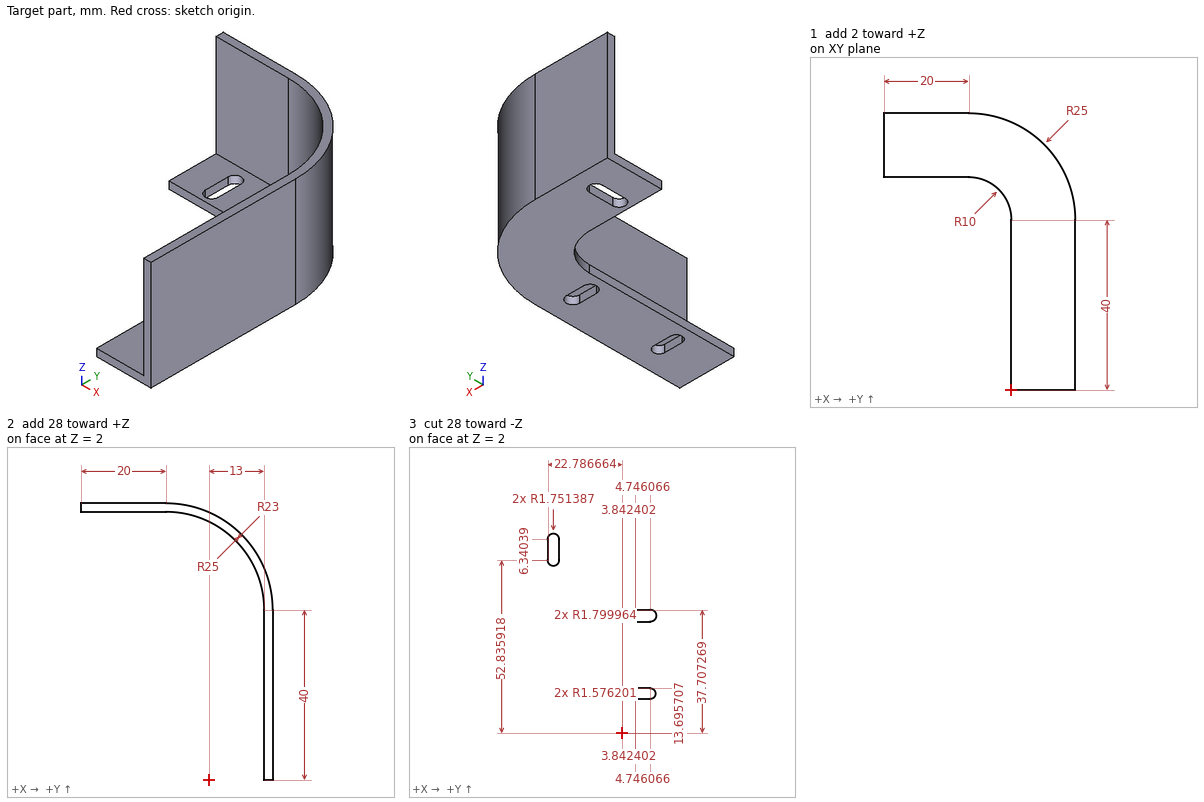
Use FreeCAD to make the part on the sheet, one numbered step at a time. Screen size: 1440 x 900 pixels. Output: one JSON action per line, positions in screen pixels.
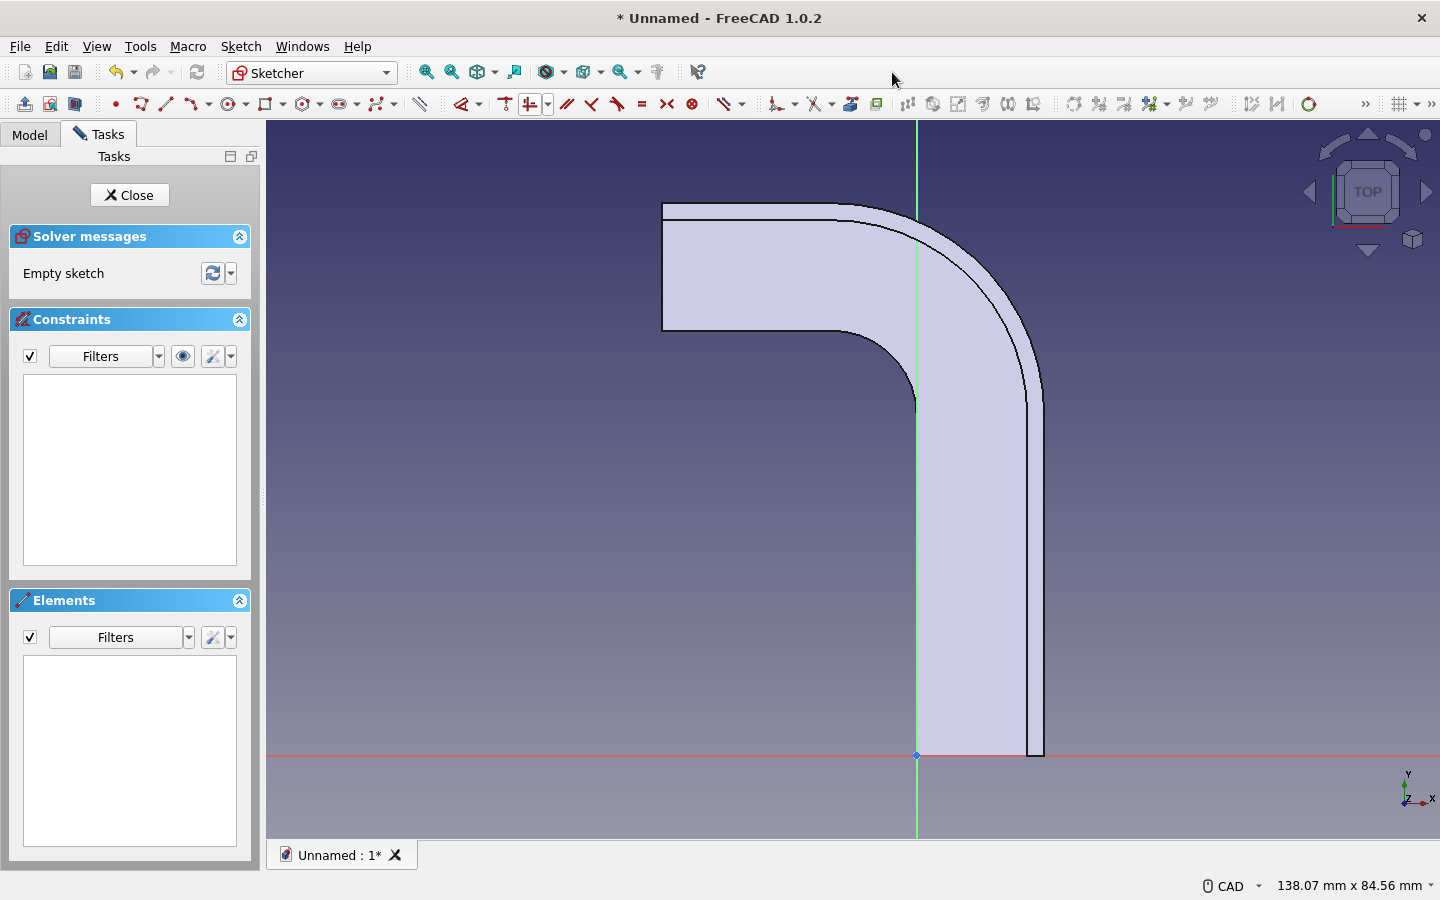
{"action": "left_click", "coordinate": [75, 104]}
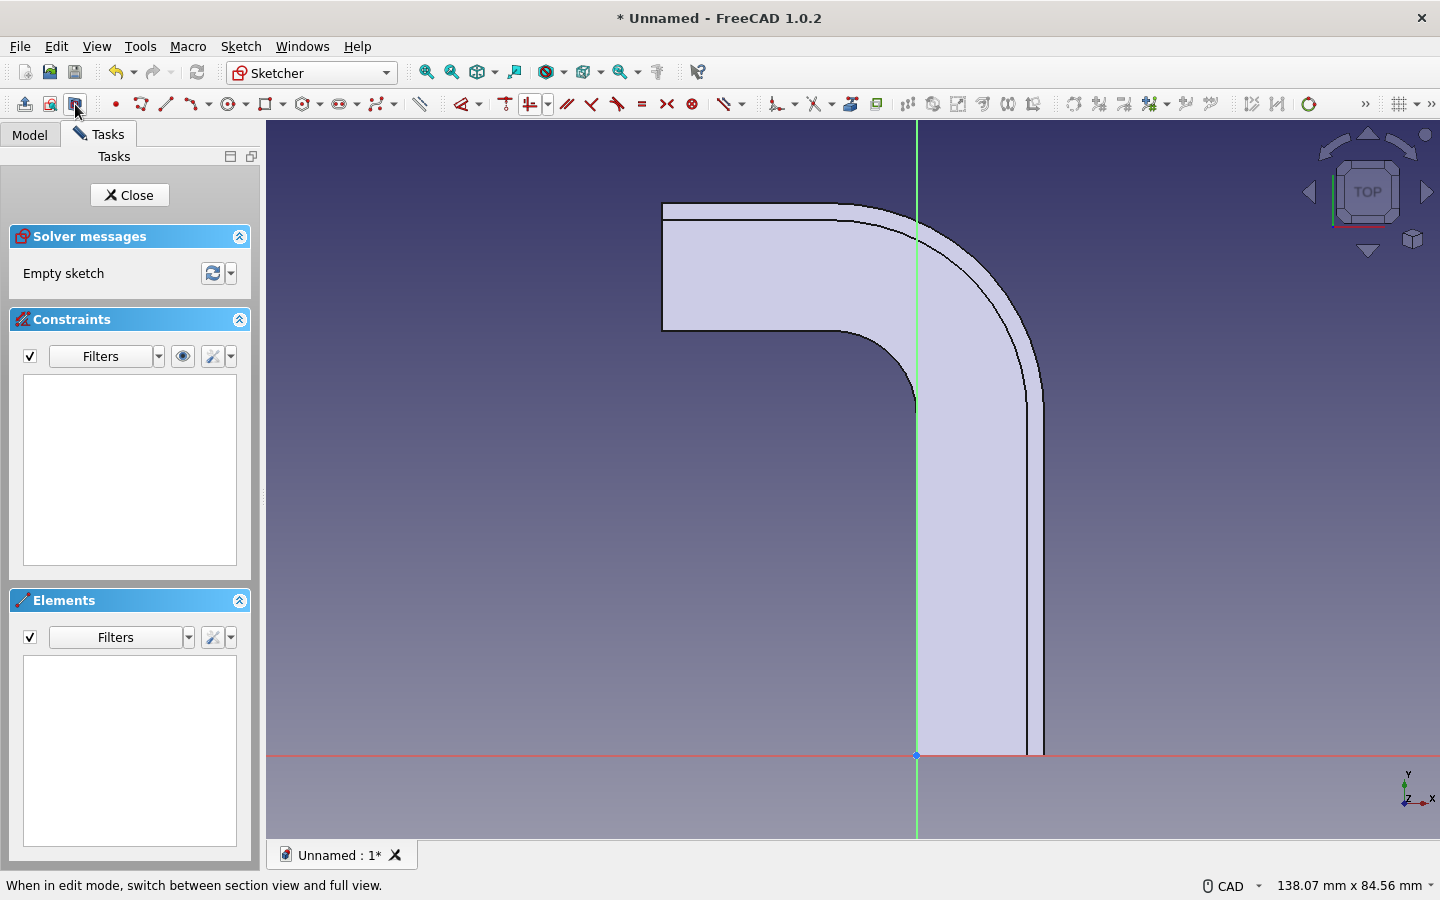
{"action": "left_click", "coordinate": [338, 104]}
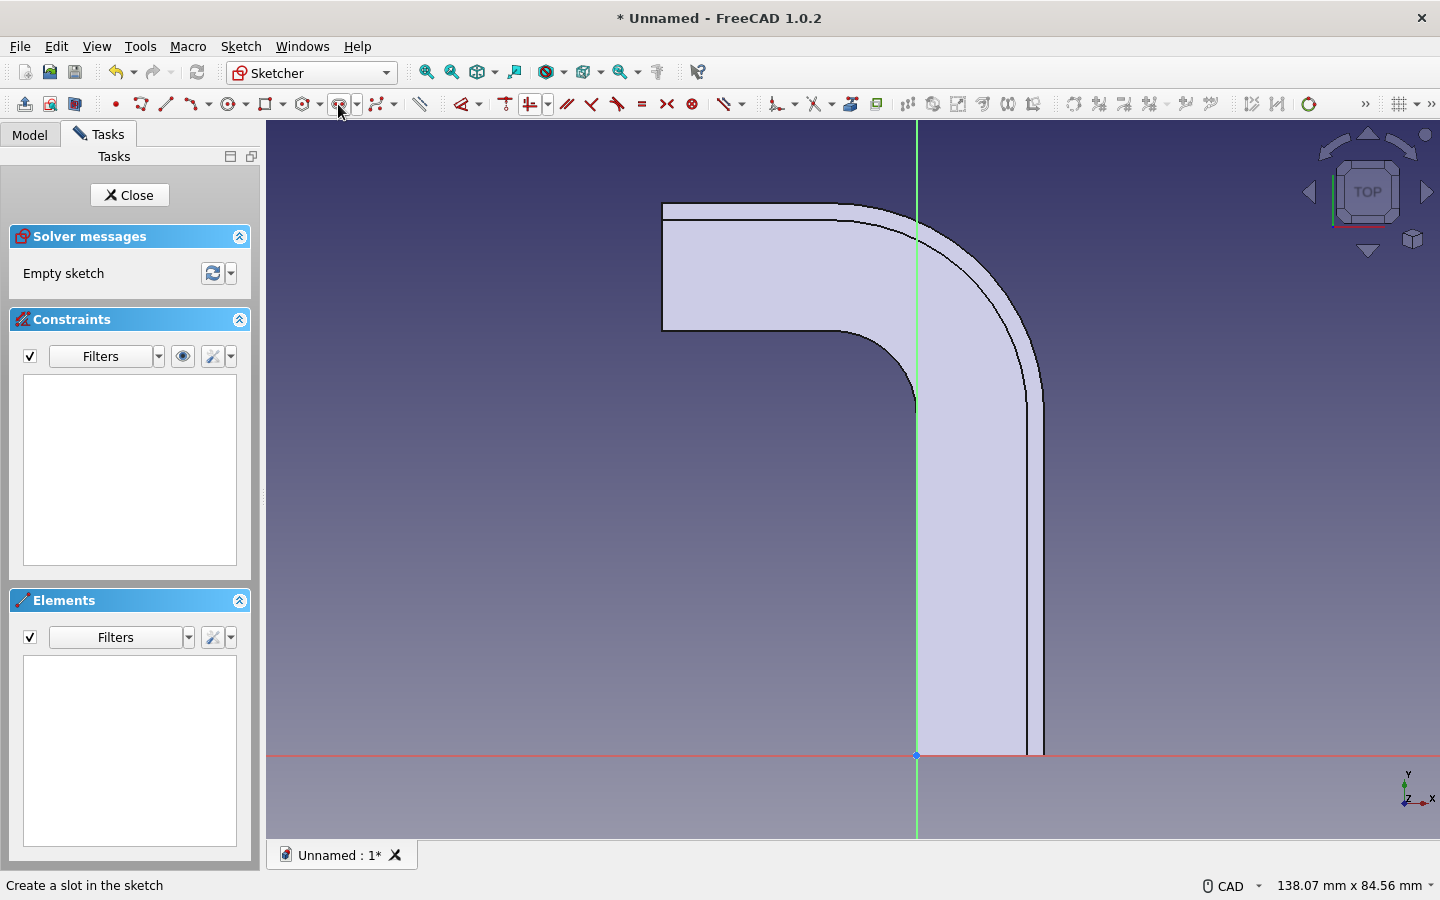
{"action": "scroll", "coordinate": [738, 307], "scroll_direction": "up", "scroll_amount": 3}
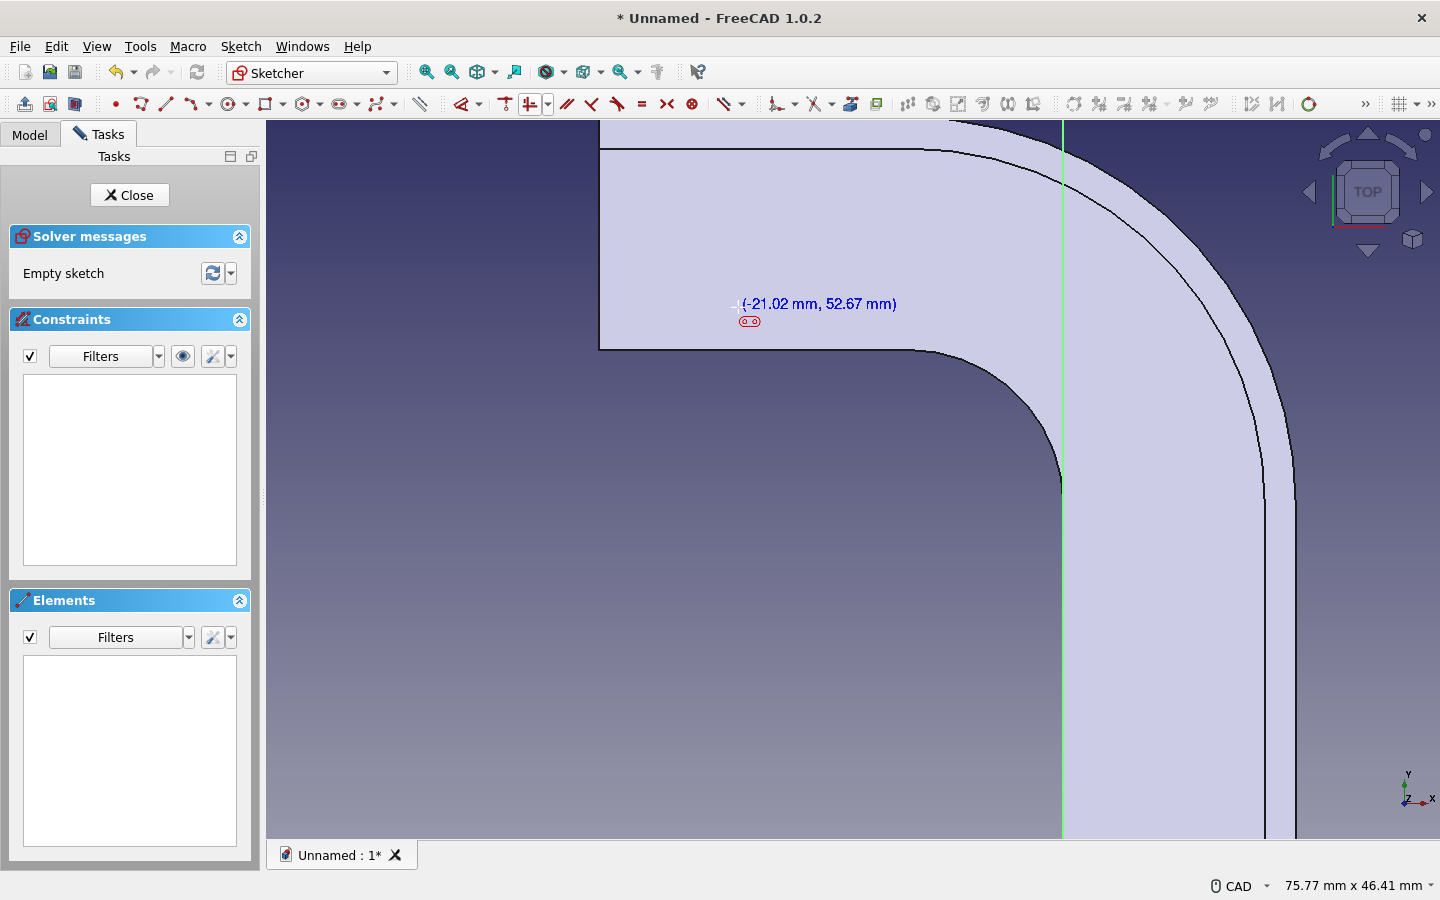
{"action": "left_click", "coordinate": [738, 306]}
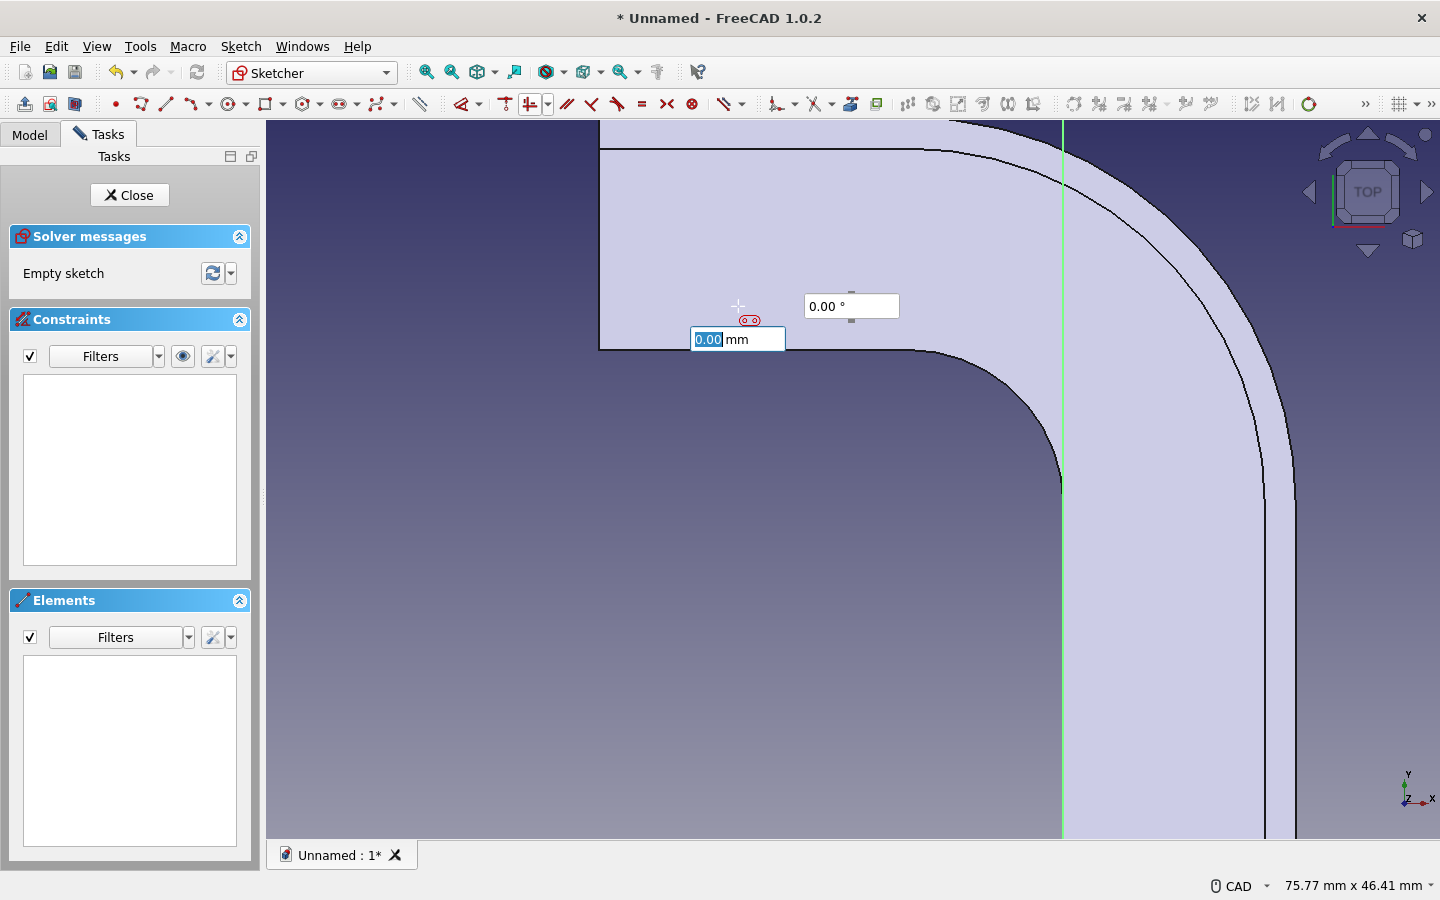
{"action": "left_click", "coordinate": [738, 208]}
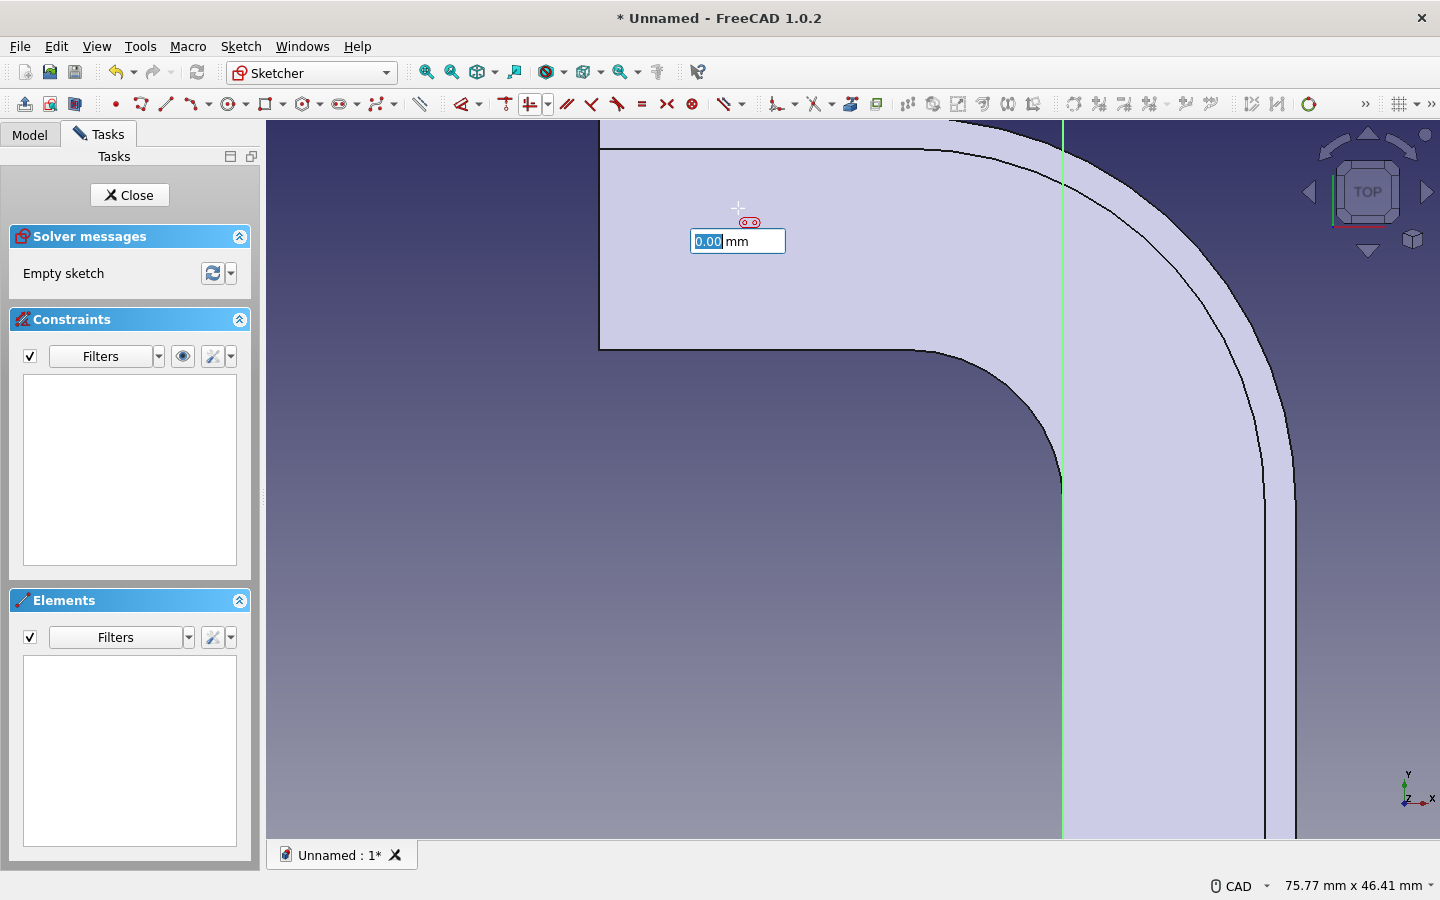
{"action": "left_click", "coordinate": [765, 257]}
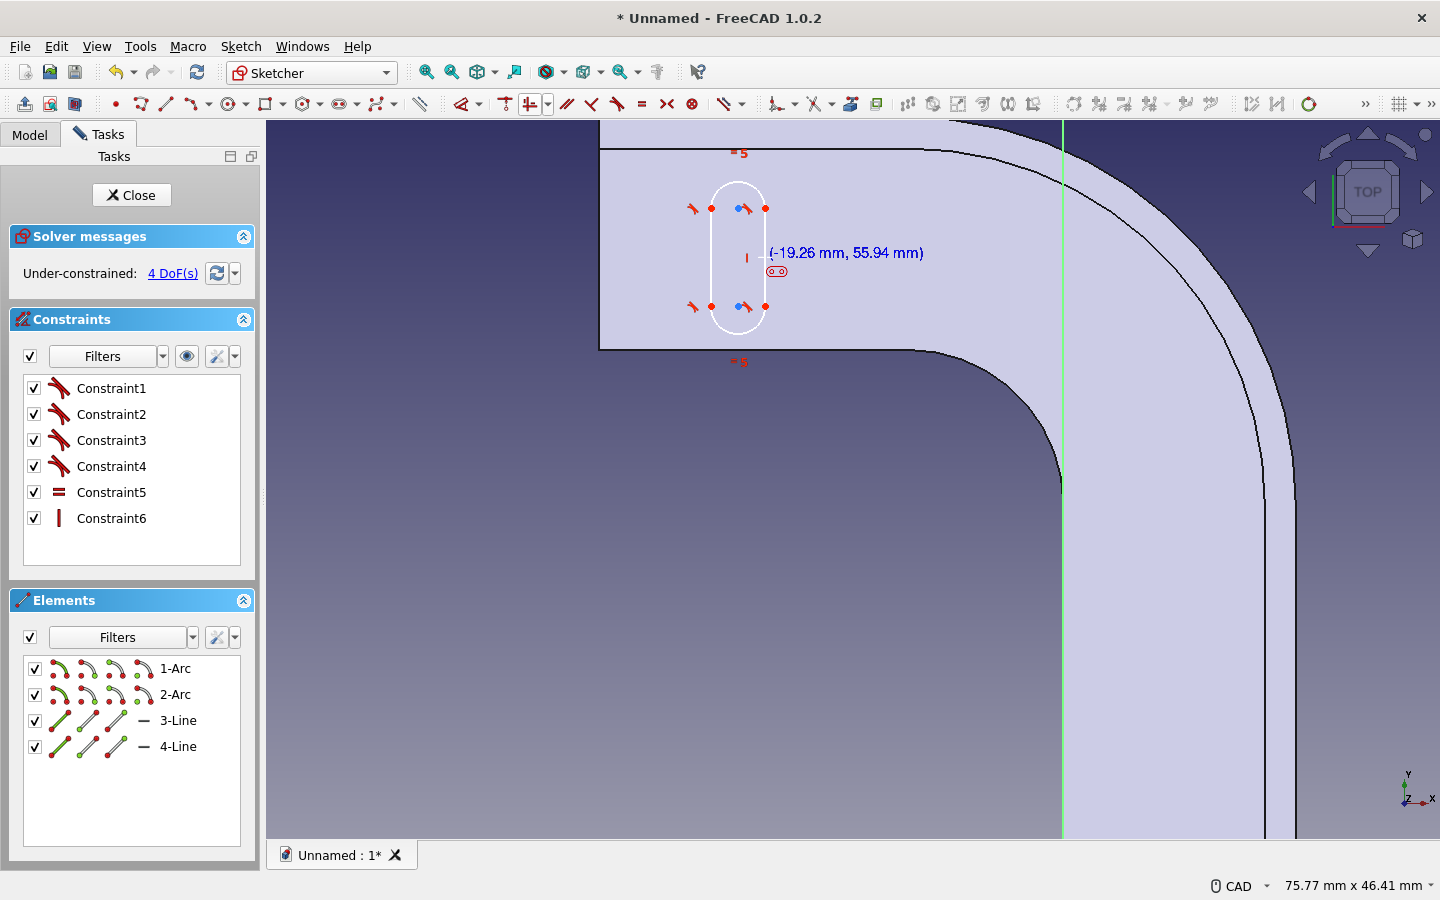
{"action": "scroll", "coordinate": [635, 338], "scroll_direction": "down", "scroll_amount": 4}